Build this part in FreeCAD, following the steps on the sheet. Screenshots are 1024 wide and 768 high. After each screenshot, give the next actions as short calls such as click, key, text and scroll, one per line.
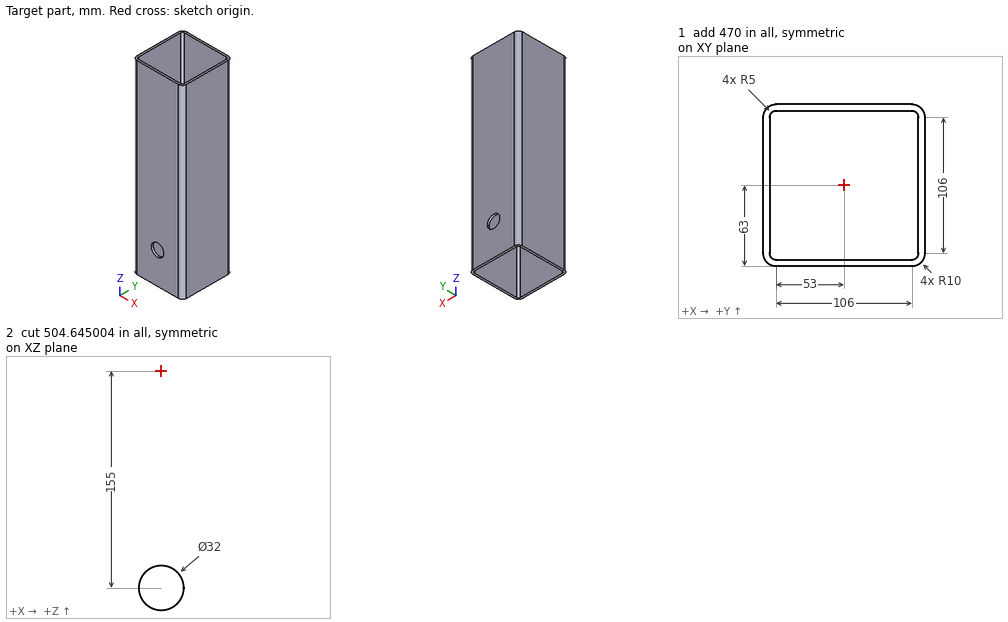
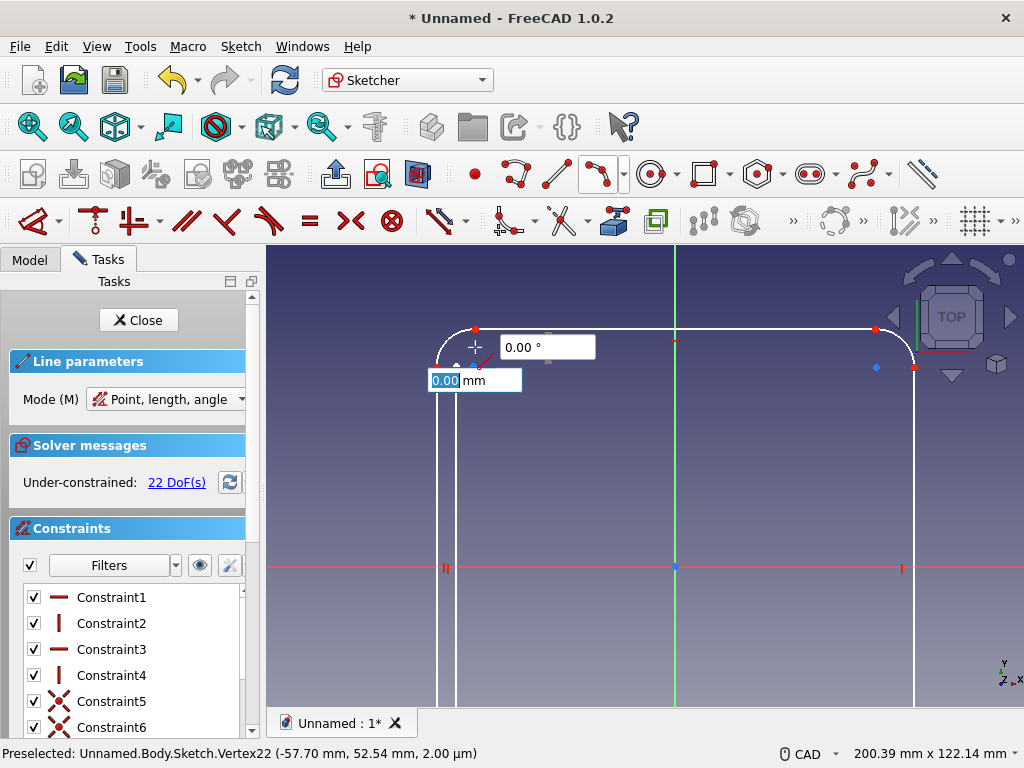
scroll(456, 366, down, 3)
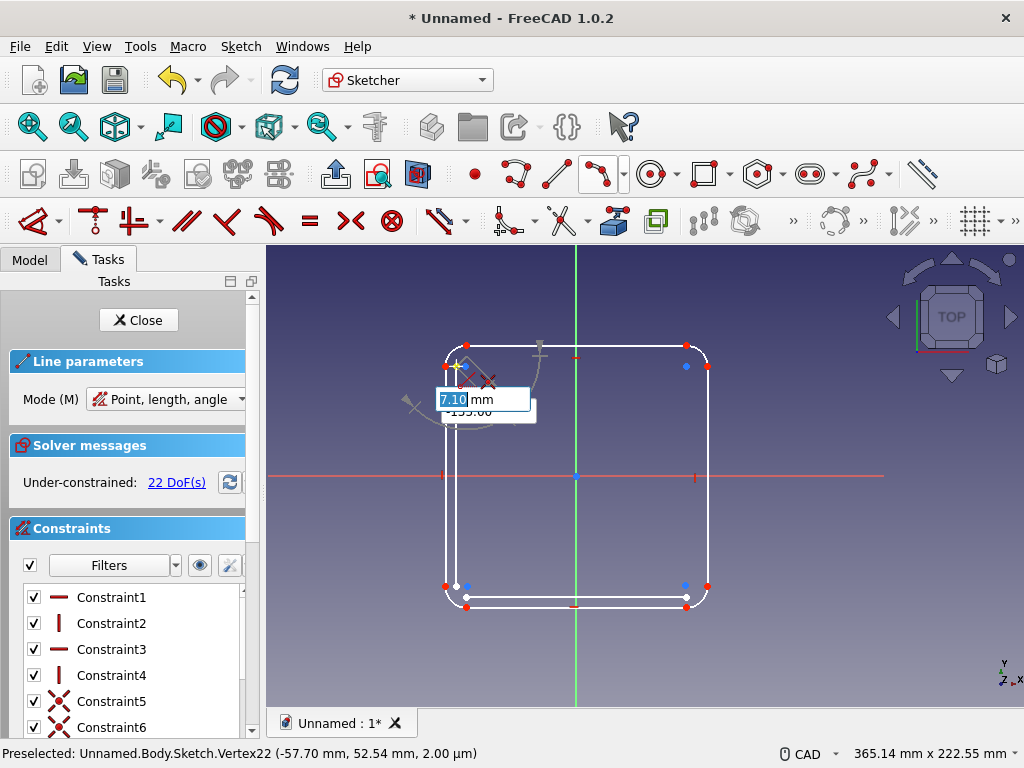
scroll(686, 356, up, 3)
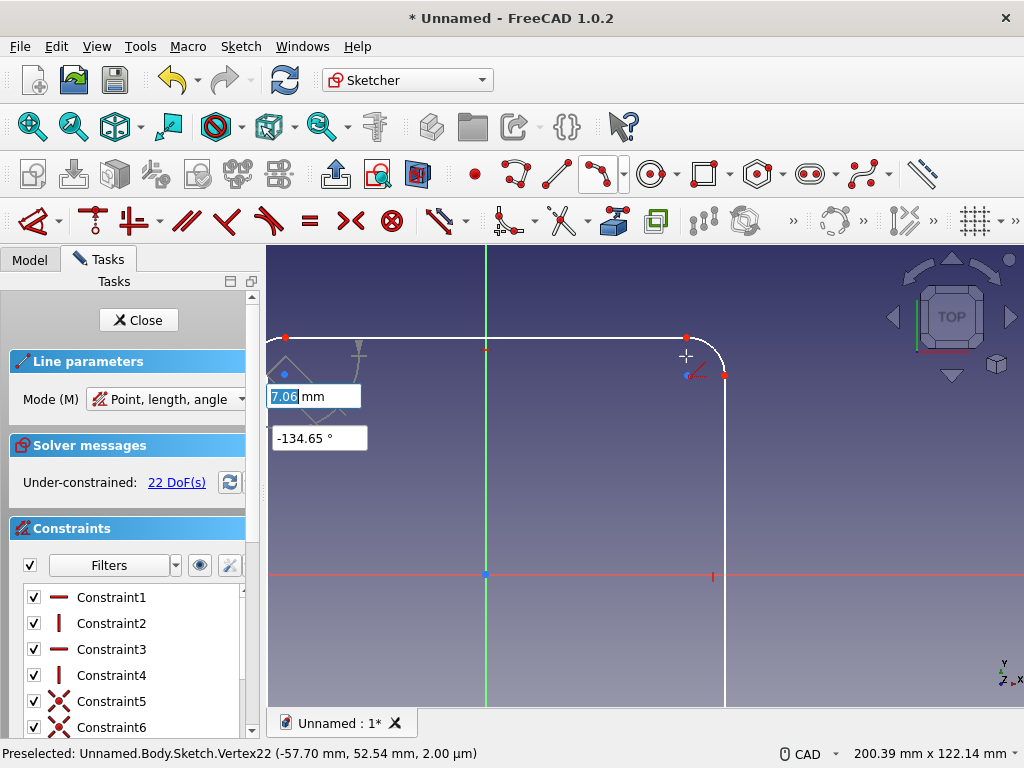
click(686, 355)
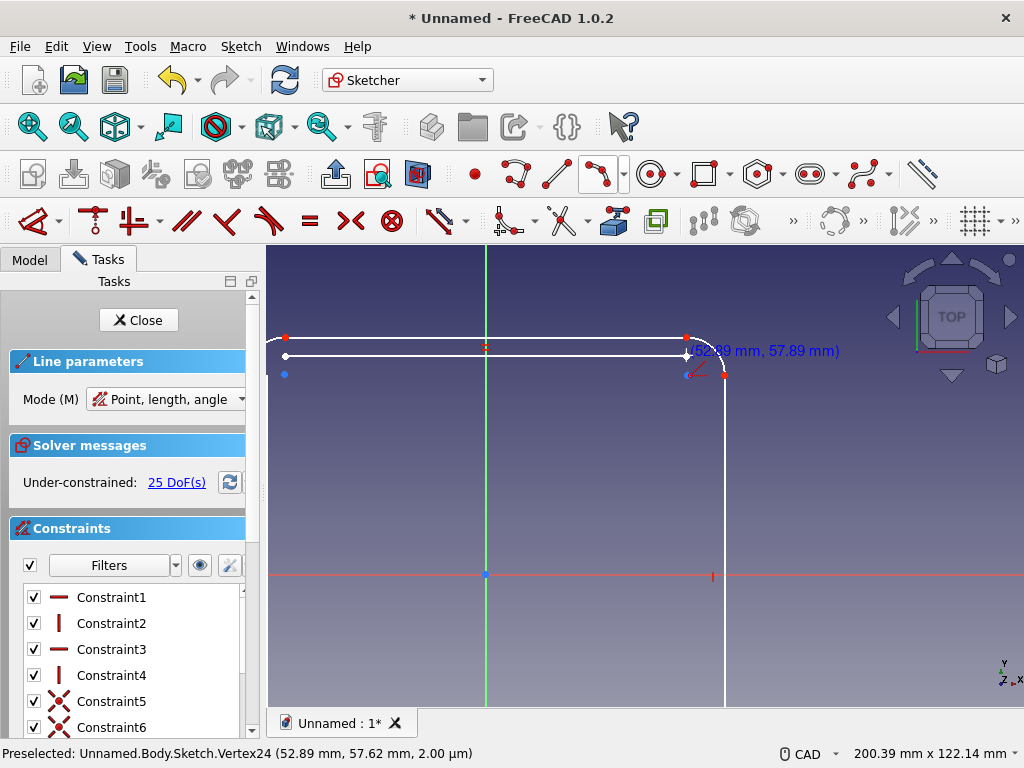
click(705, 374)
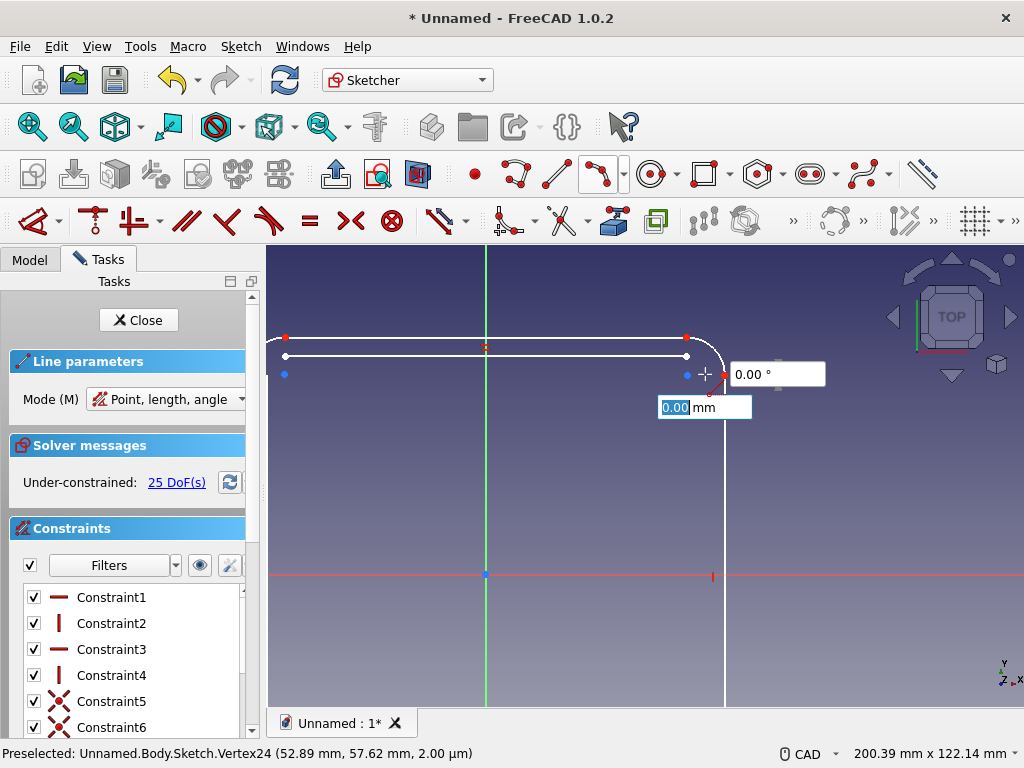
scroll(687, 356, down, 3)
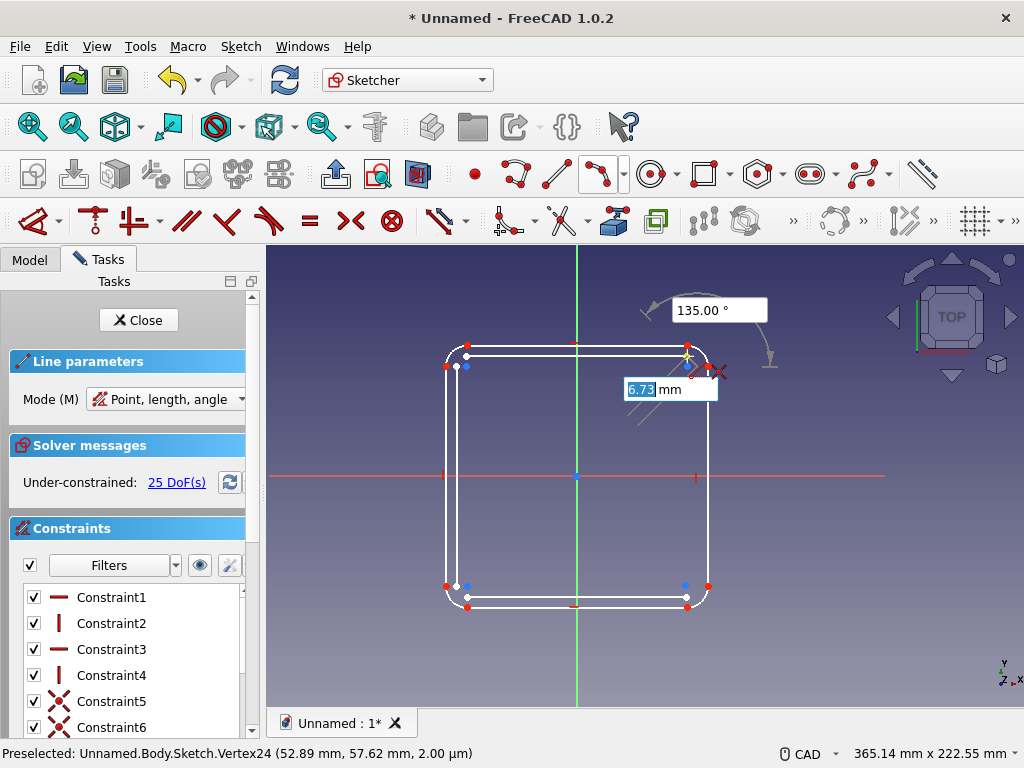
scroll(697, 586, up, 3)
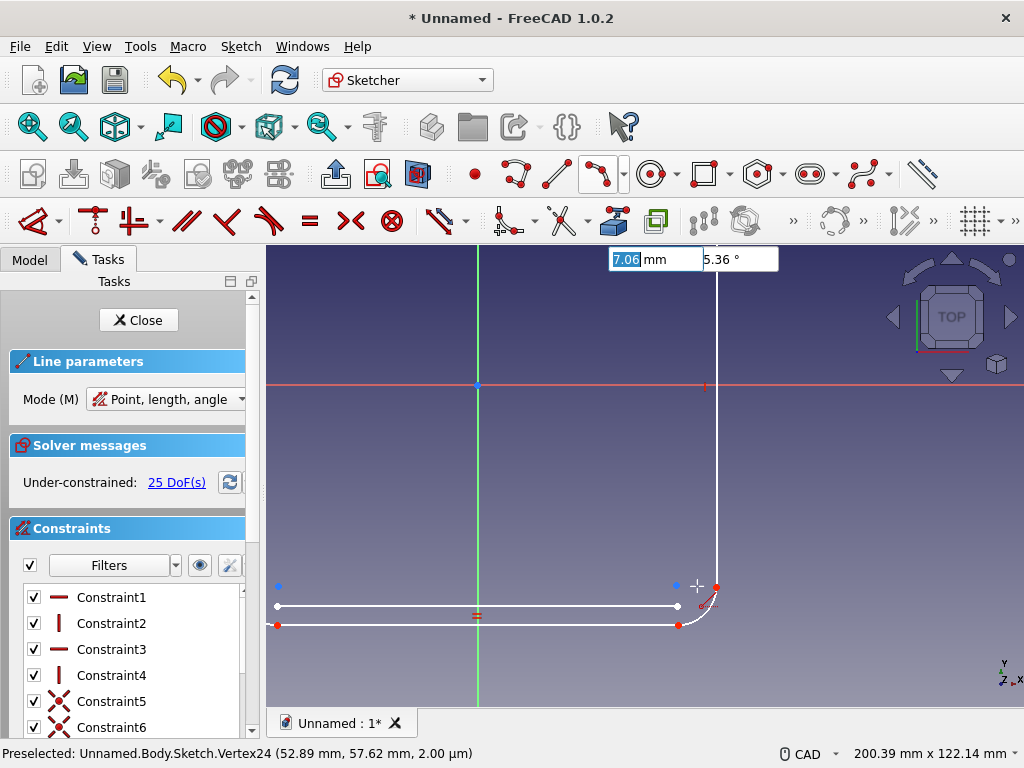
click(697, 586)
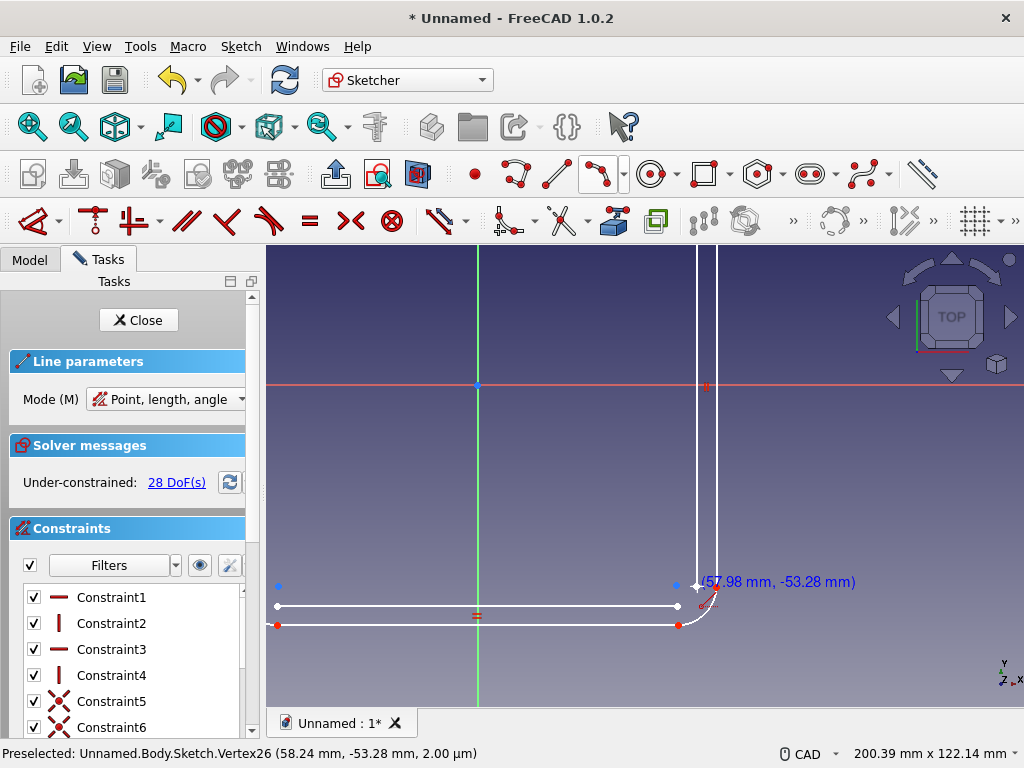
click(598, 174)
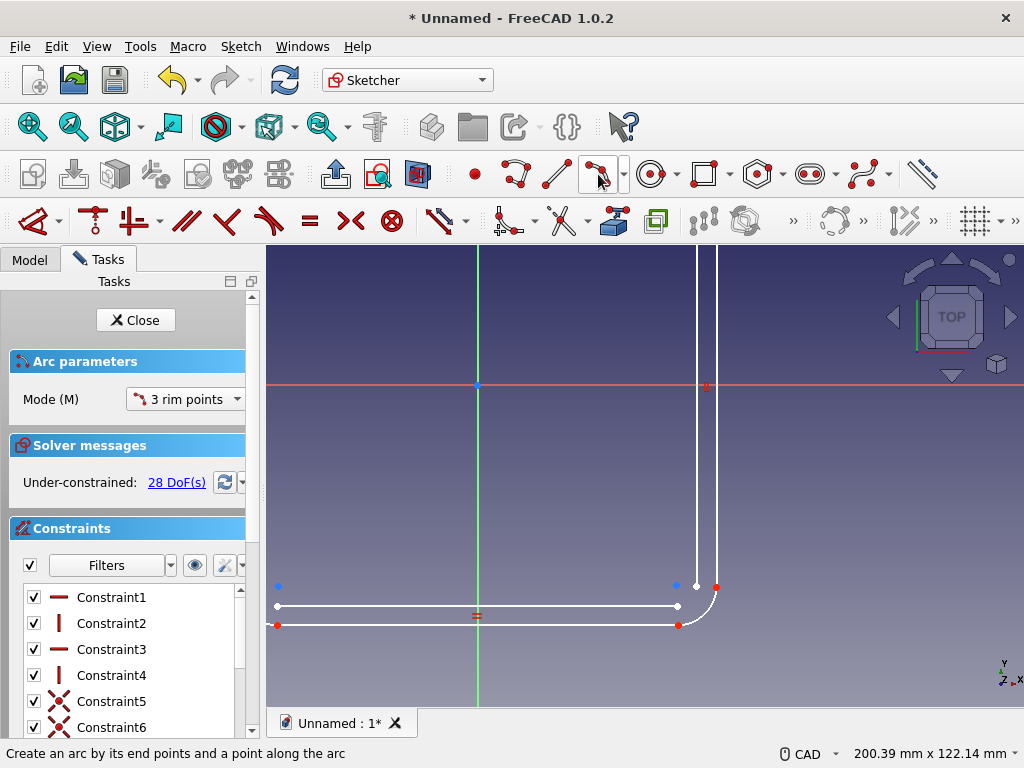
scroll(697, 586, down, 3)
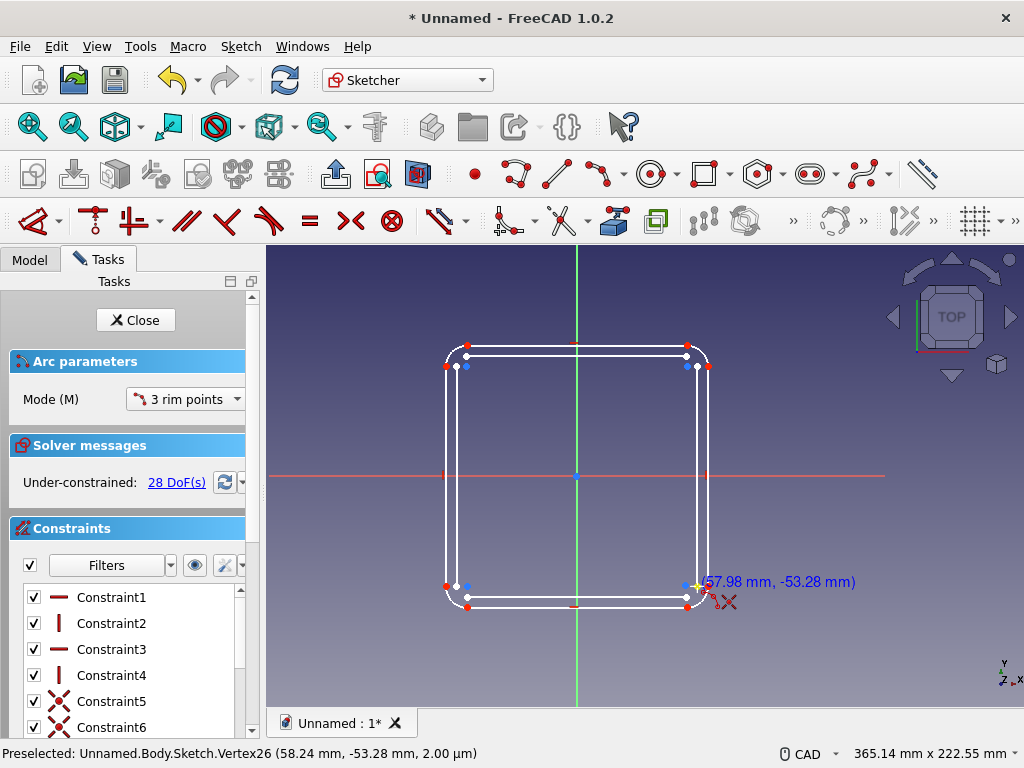
scroll(467, 597, up, 3)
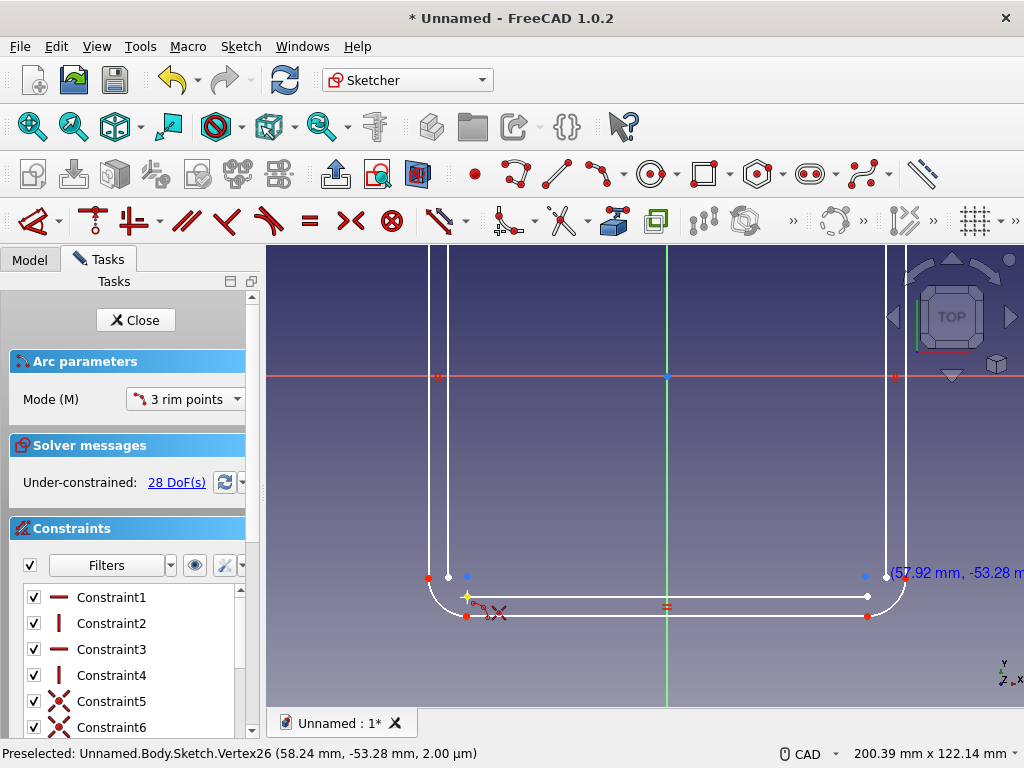
click(467, 597)
click(448, 578)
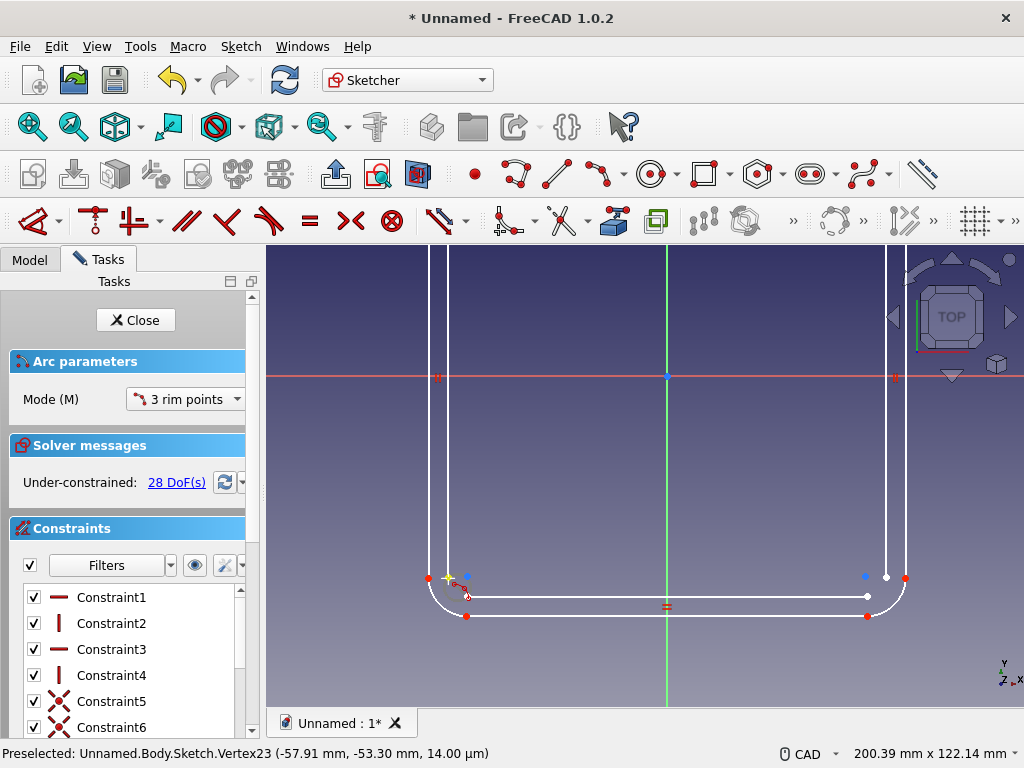
scroll(453, 590, up, 6)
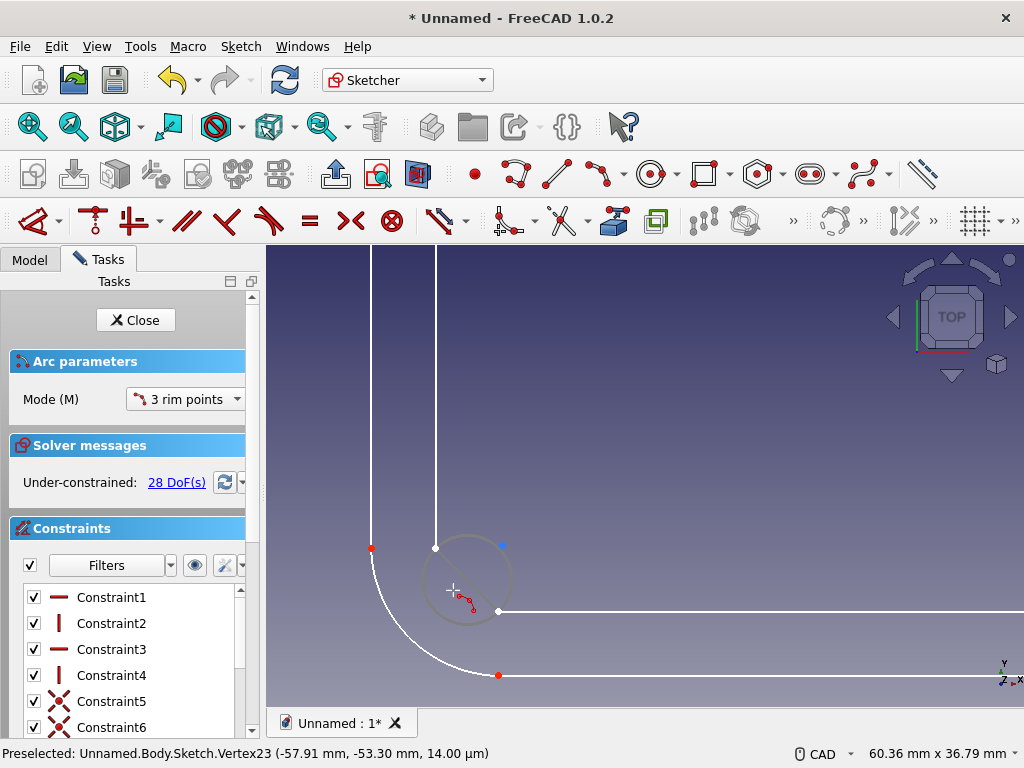
click(453, 589)